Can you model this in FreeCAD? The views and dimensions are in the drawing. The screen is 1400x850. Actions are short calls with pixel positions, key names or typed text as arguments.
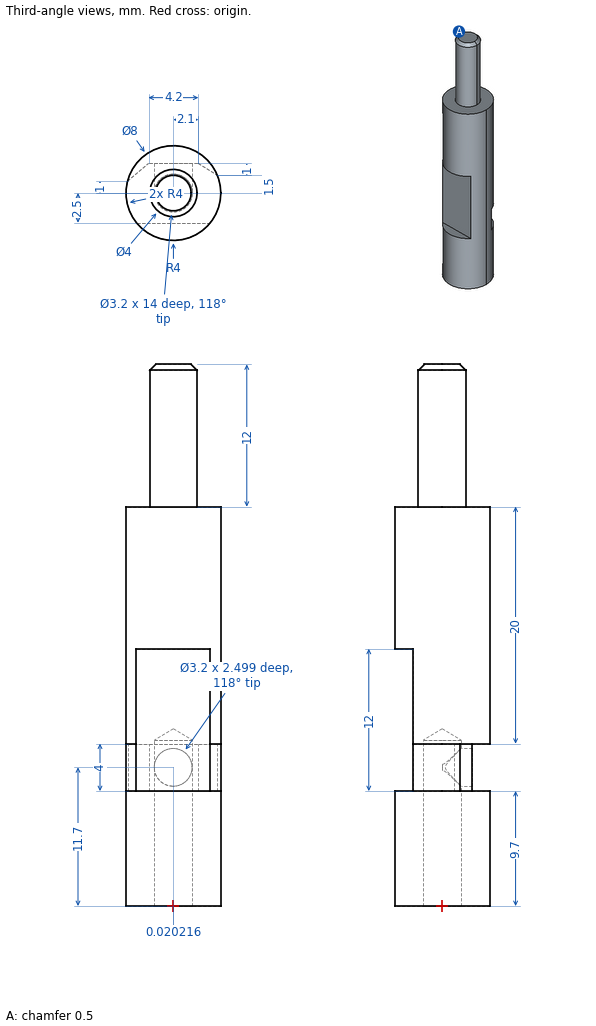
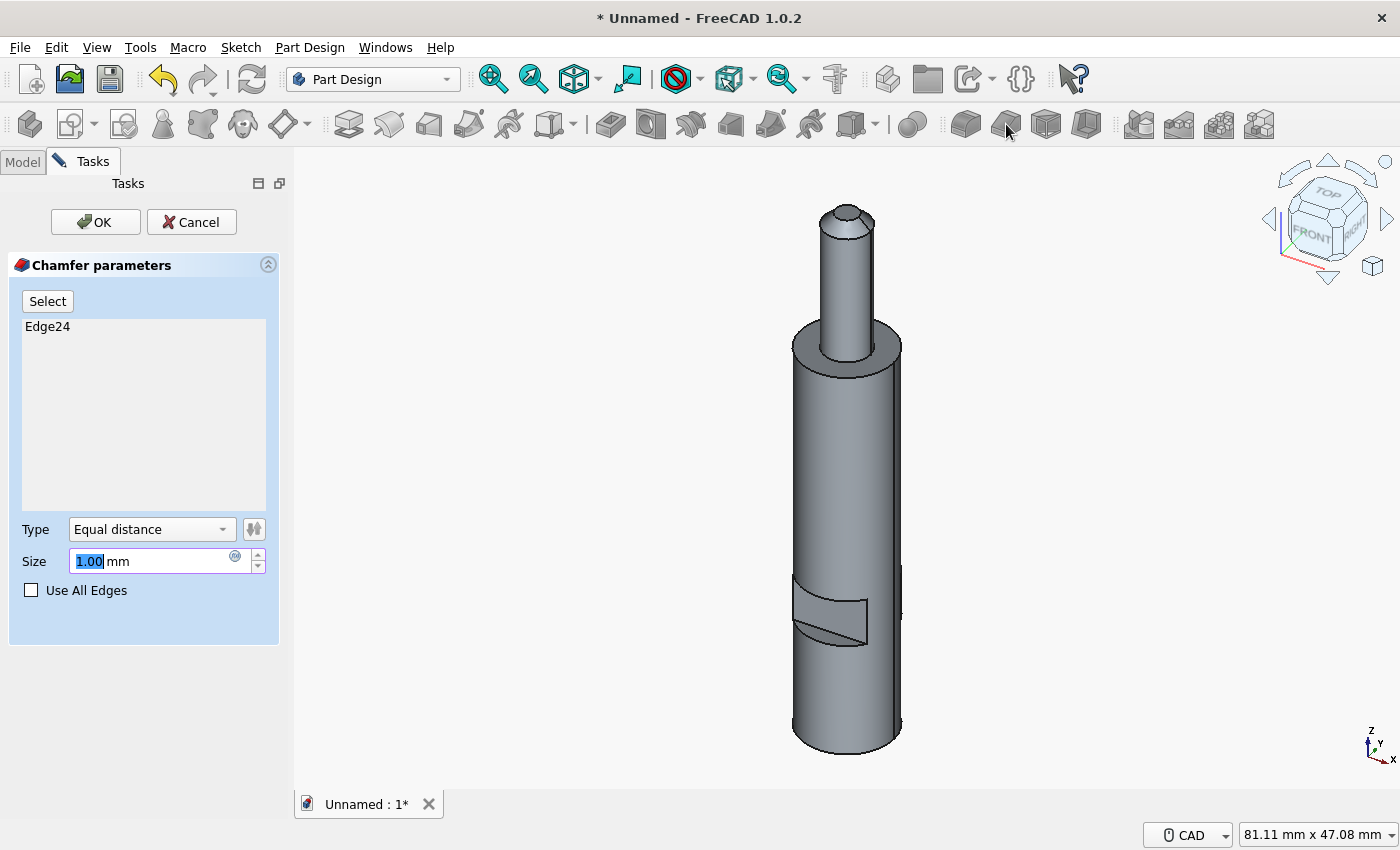
text(0.5)
key(Tab)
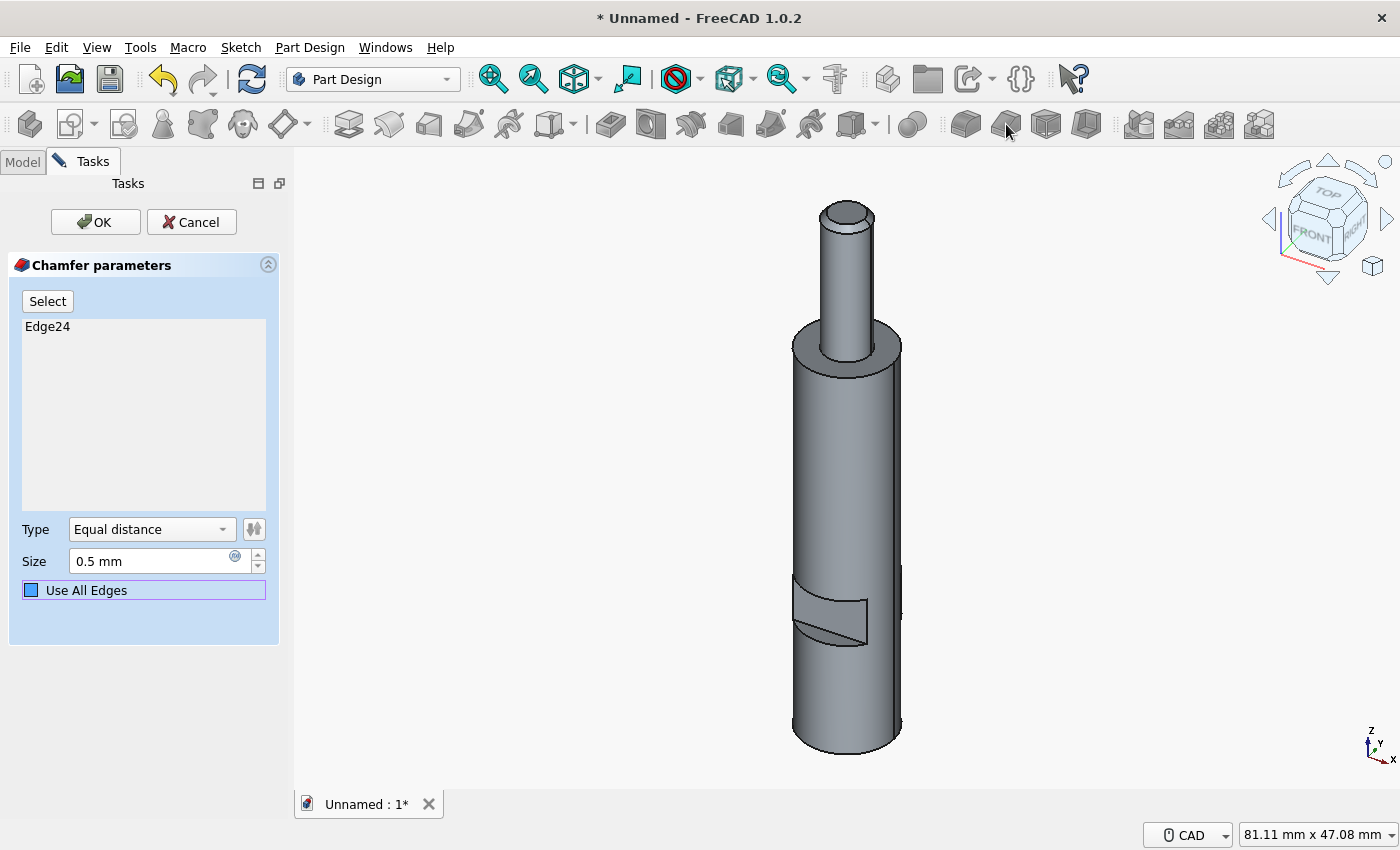
click(96, 222)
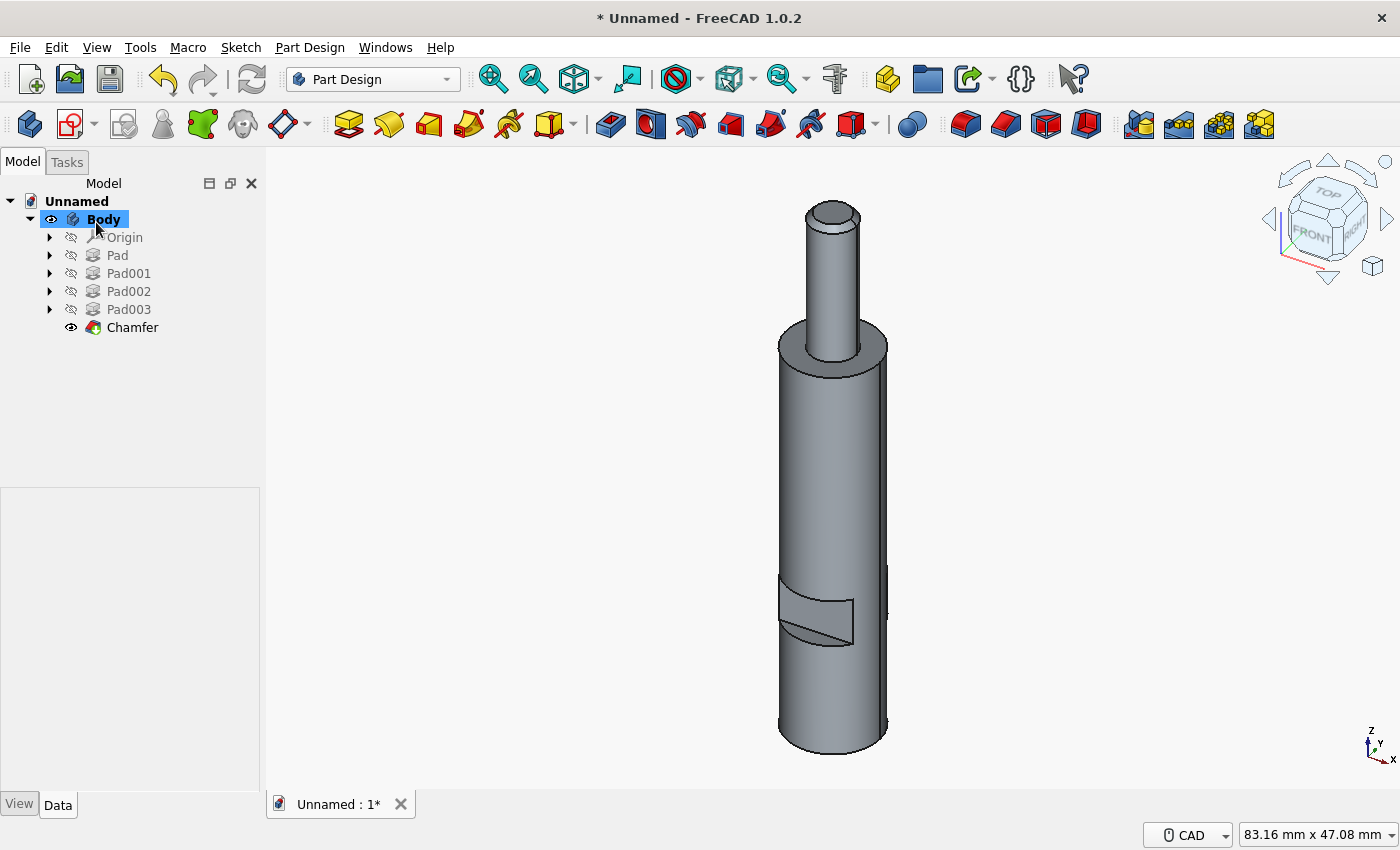
click(50, 237)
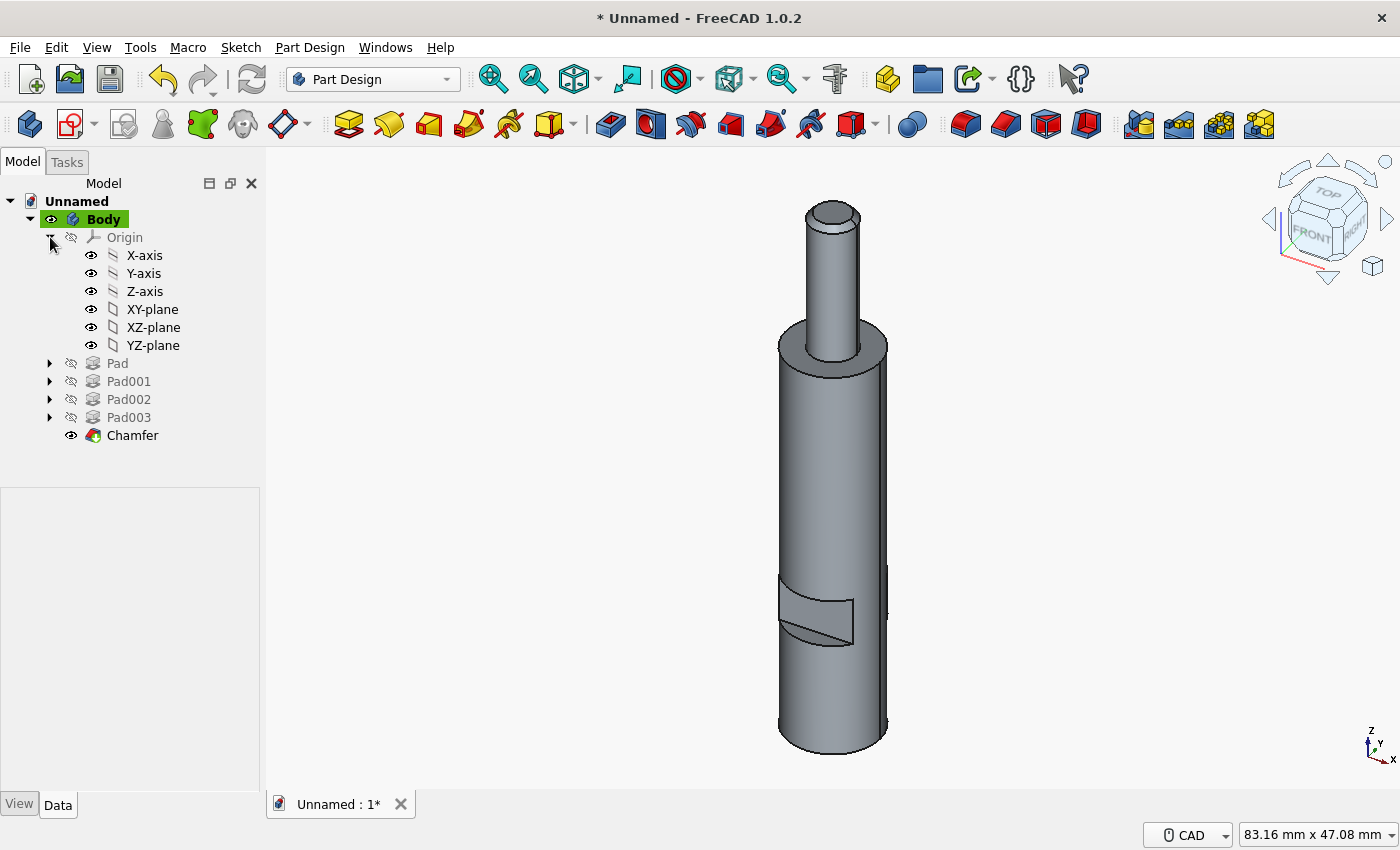
click(136, 309)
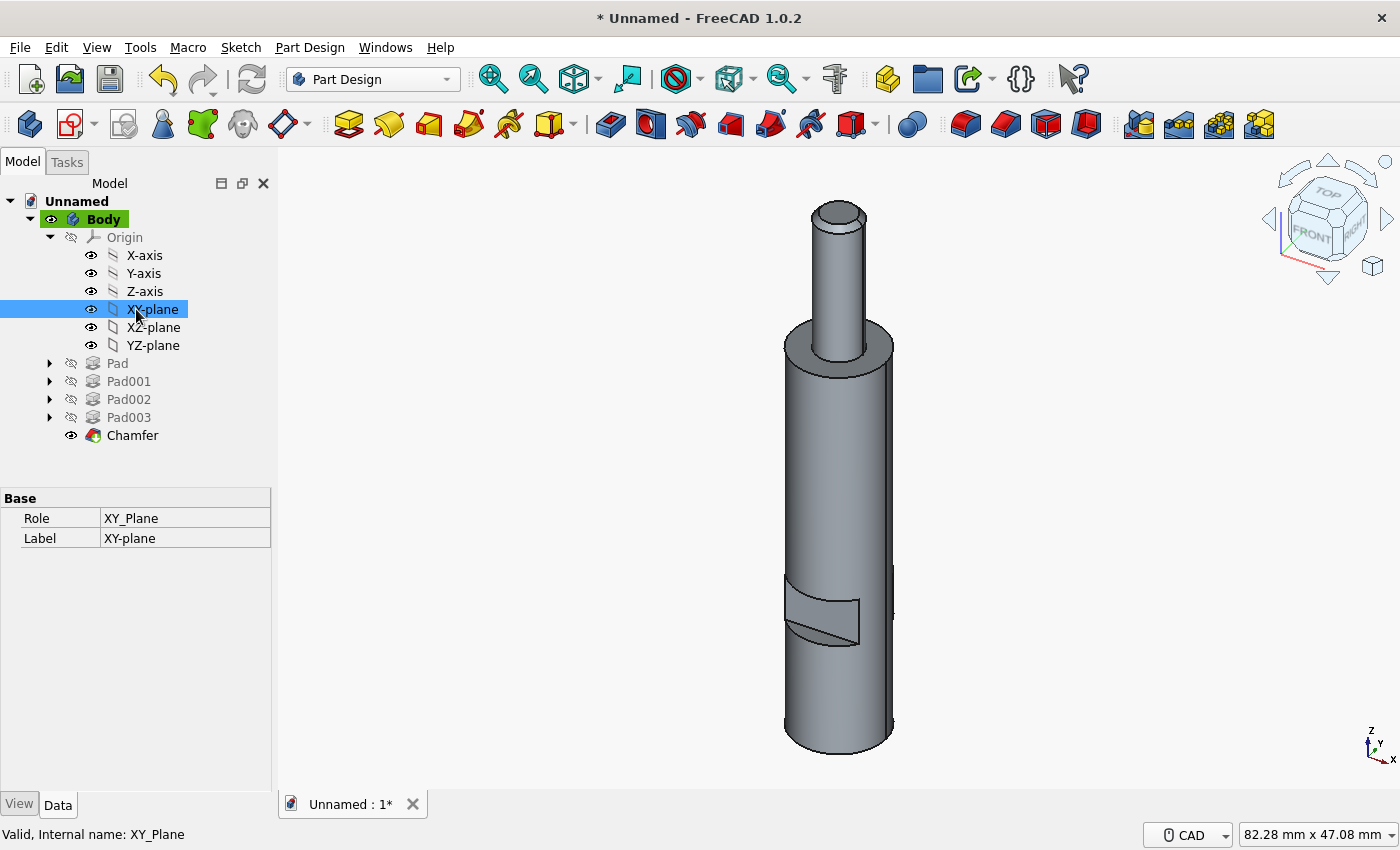
click(284, 124)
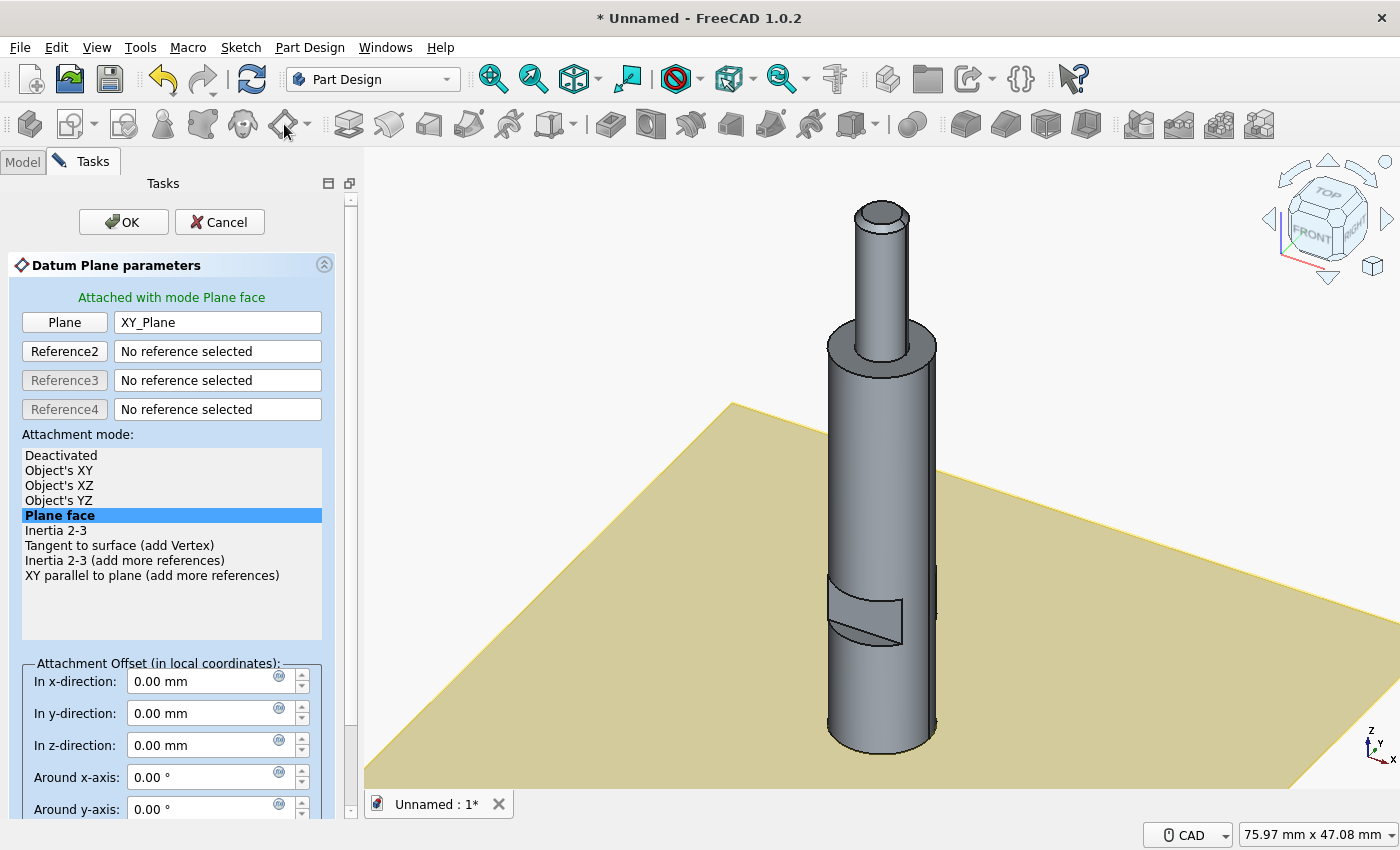
triple_click(210, 745)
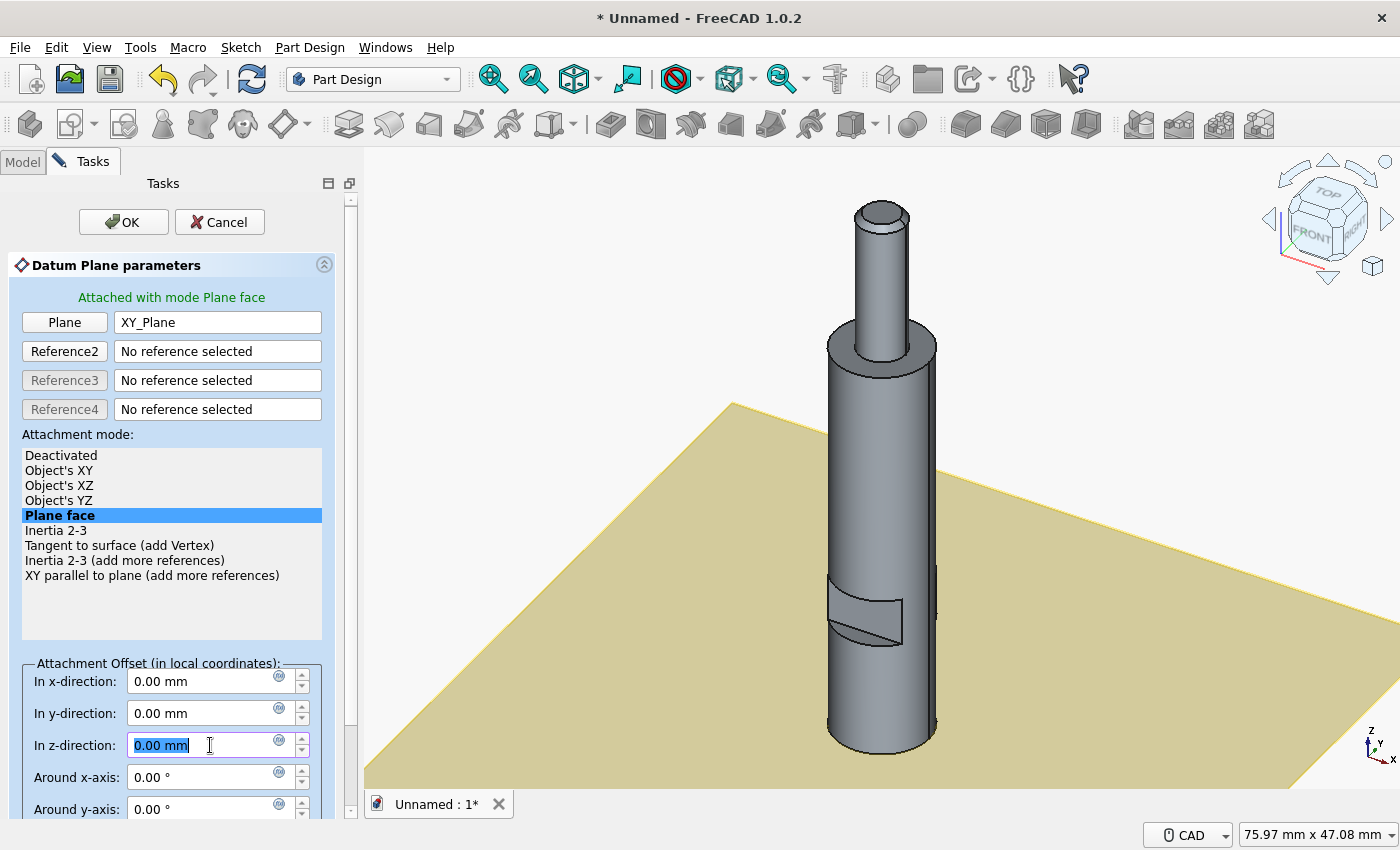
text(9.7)
key(Tab)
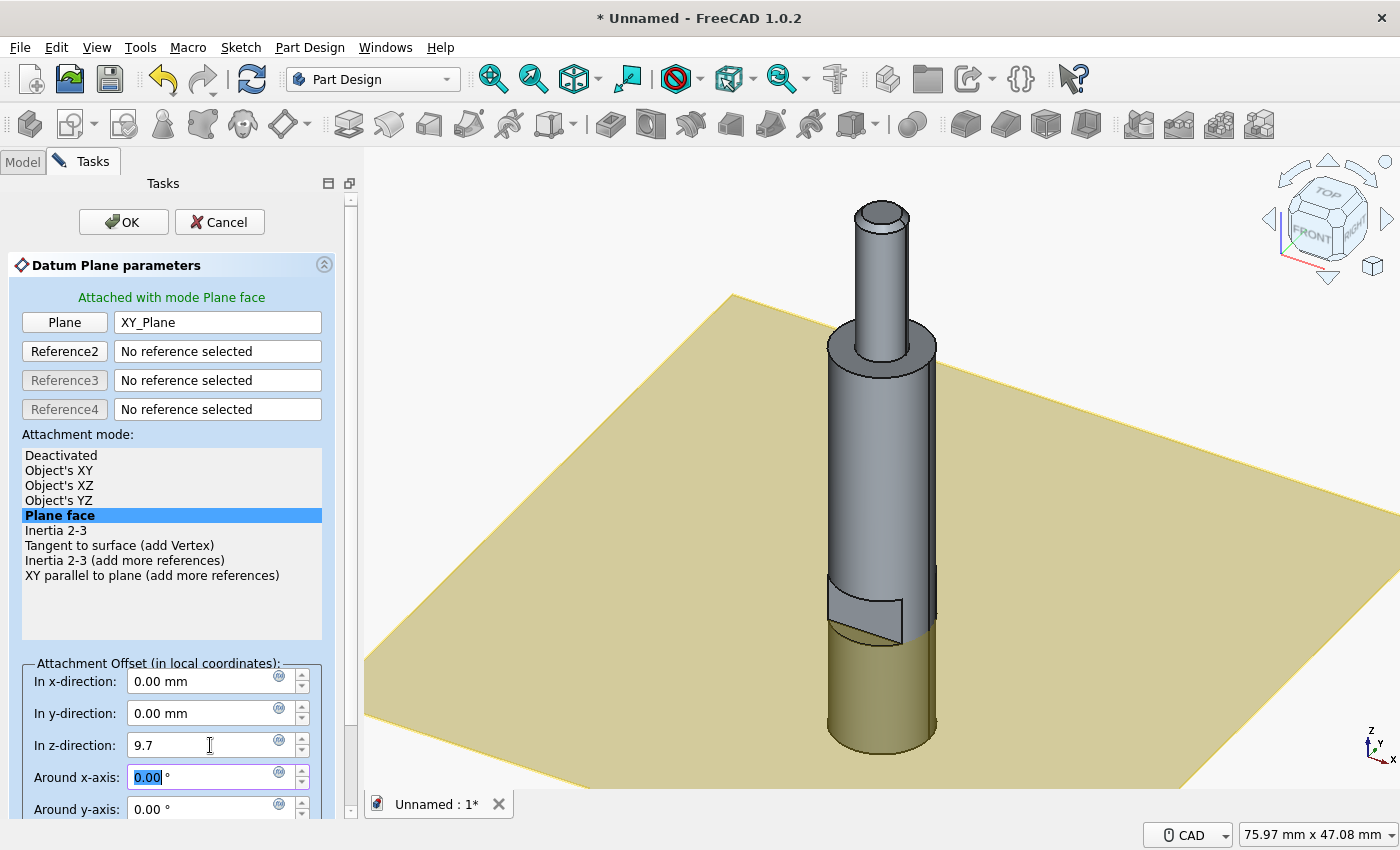
click(124, 222)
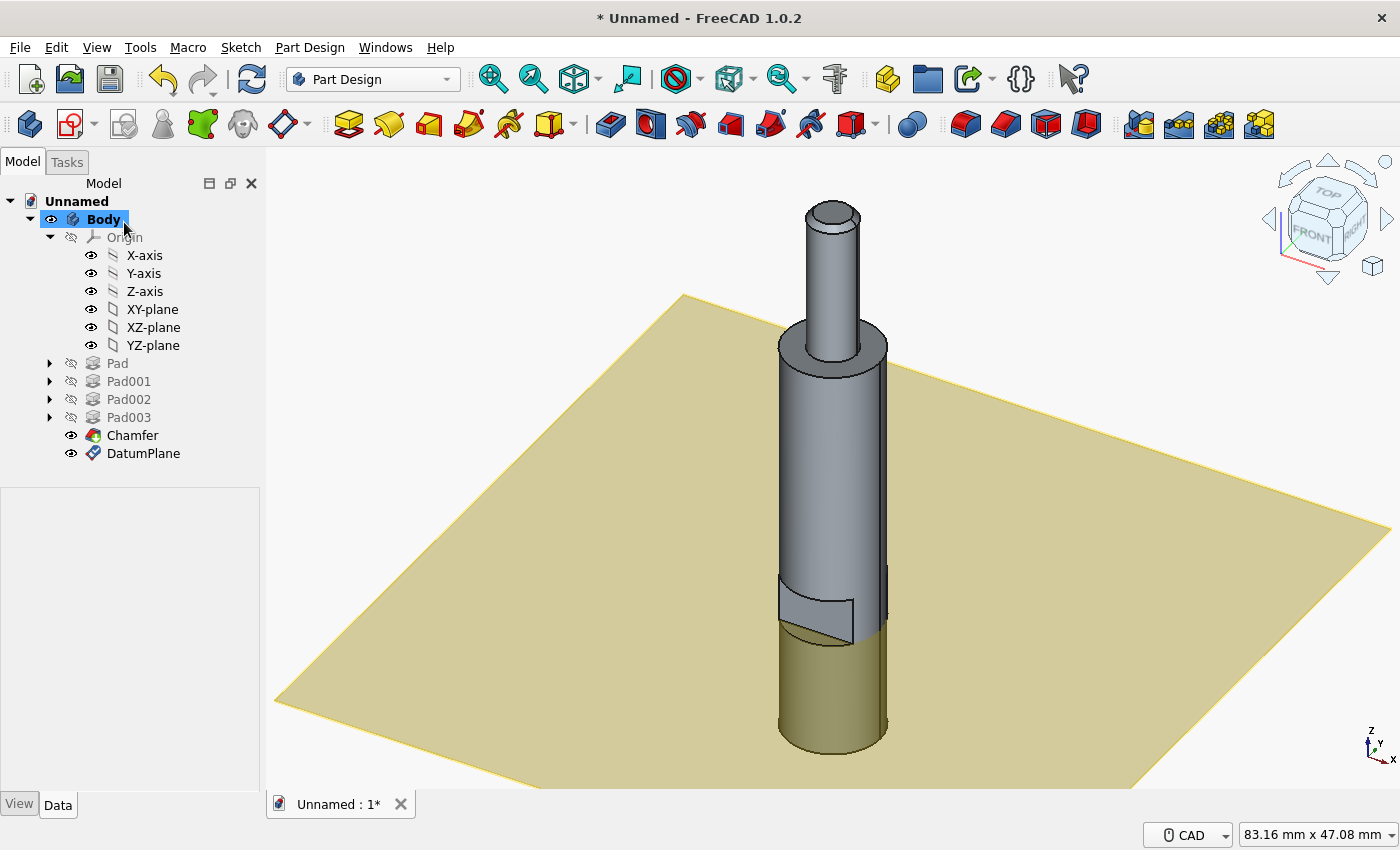
click(116, 453)